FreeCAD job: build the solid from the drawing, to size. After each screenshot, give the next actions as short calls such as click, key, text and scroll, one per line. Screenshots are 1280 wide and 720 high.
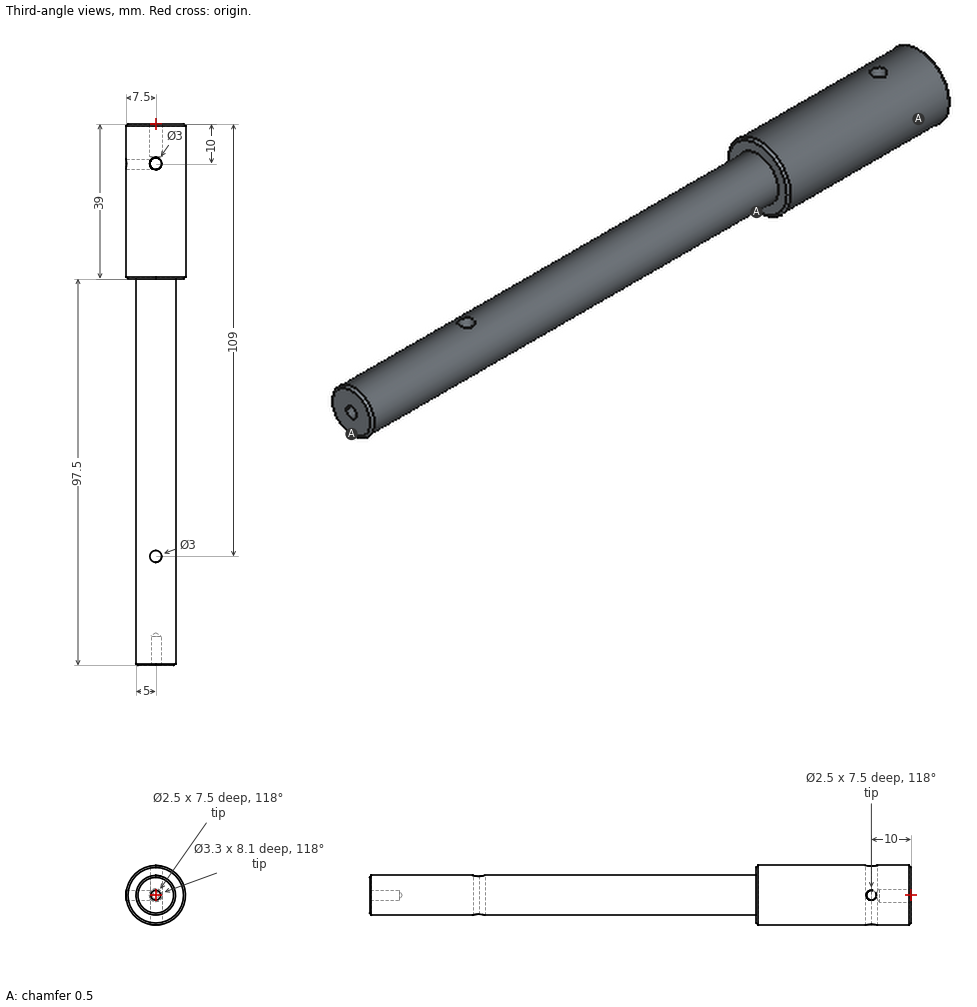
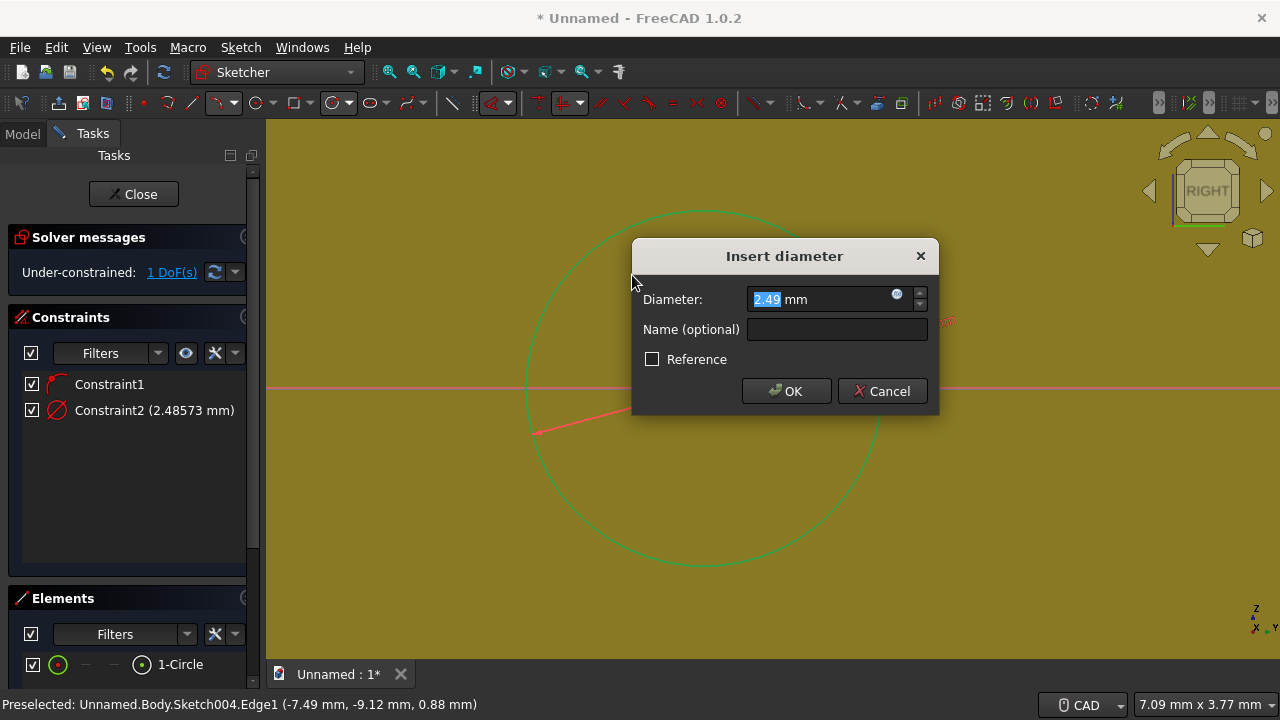
text(2.5)
key(Return)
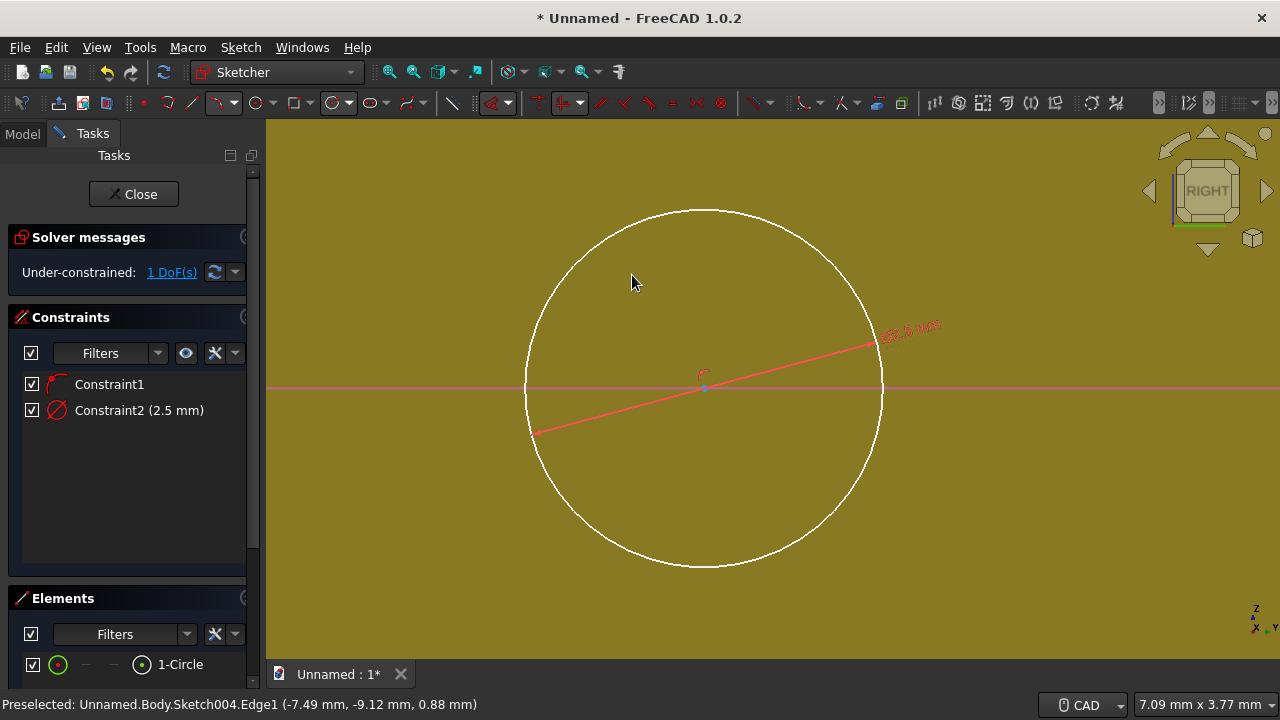
click(704, 388)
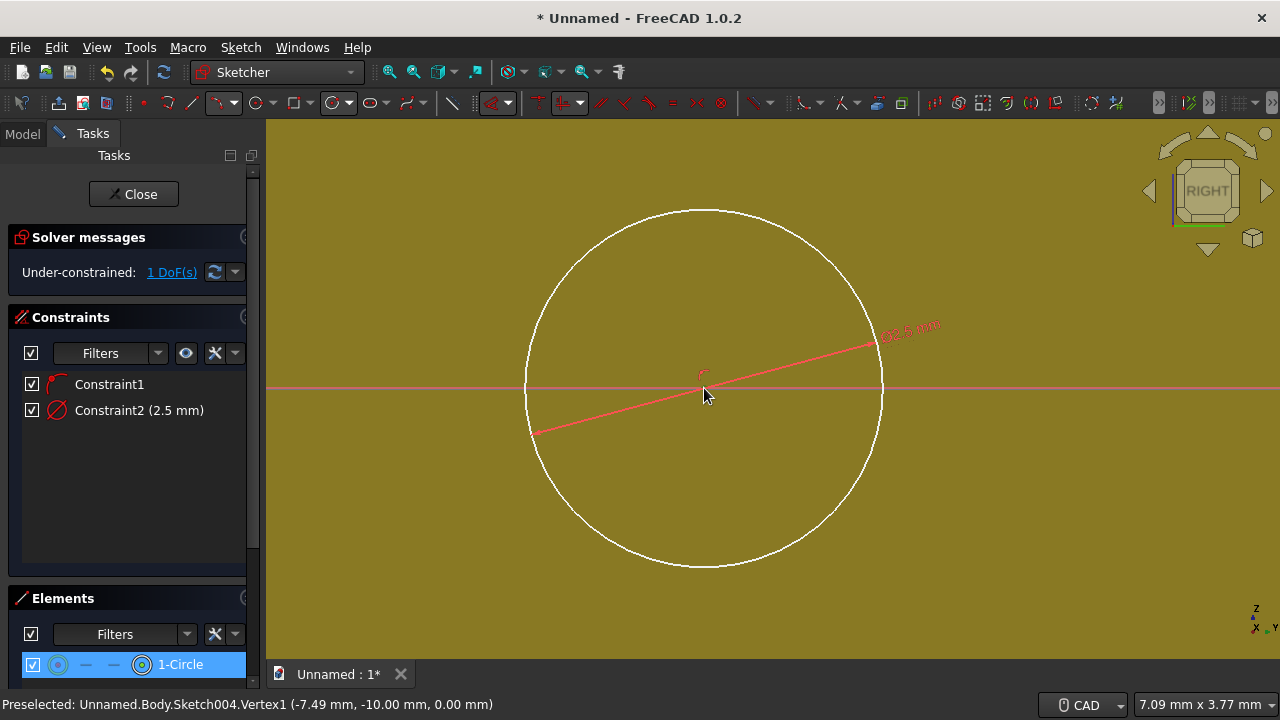
key(l)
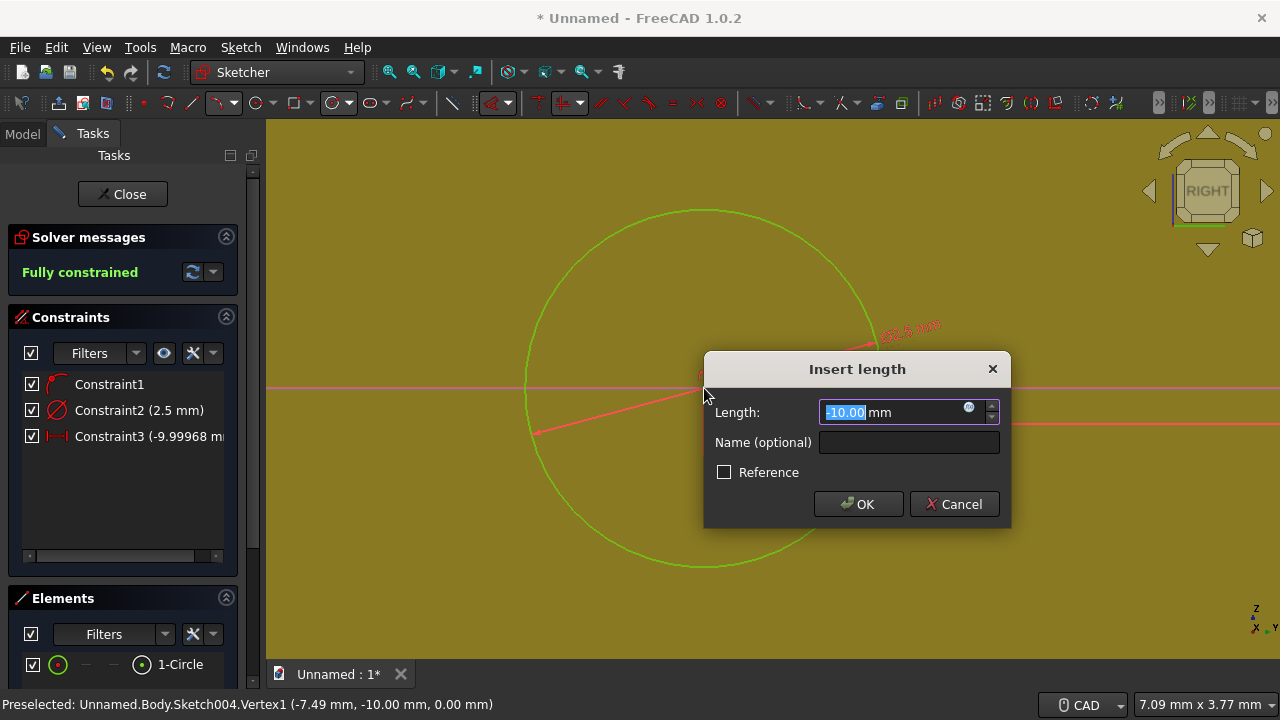
text(-10)
key(Return)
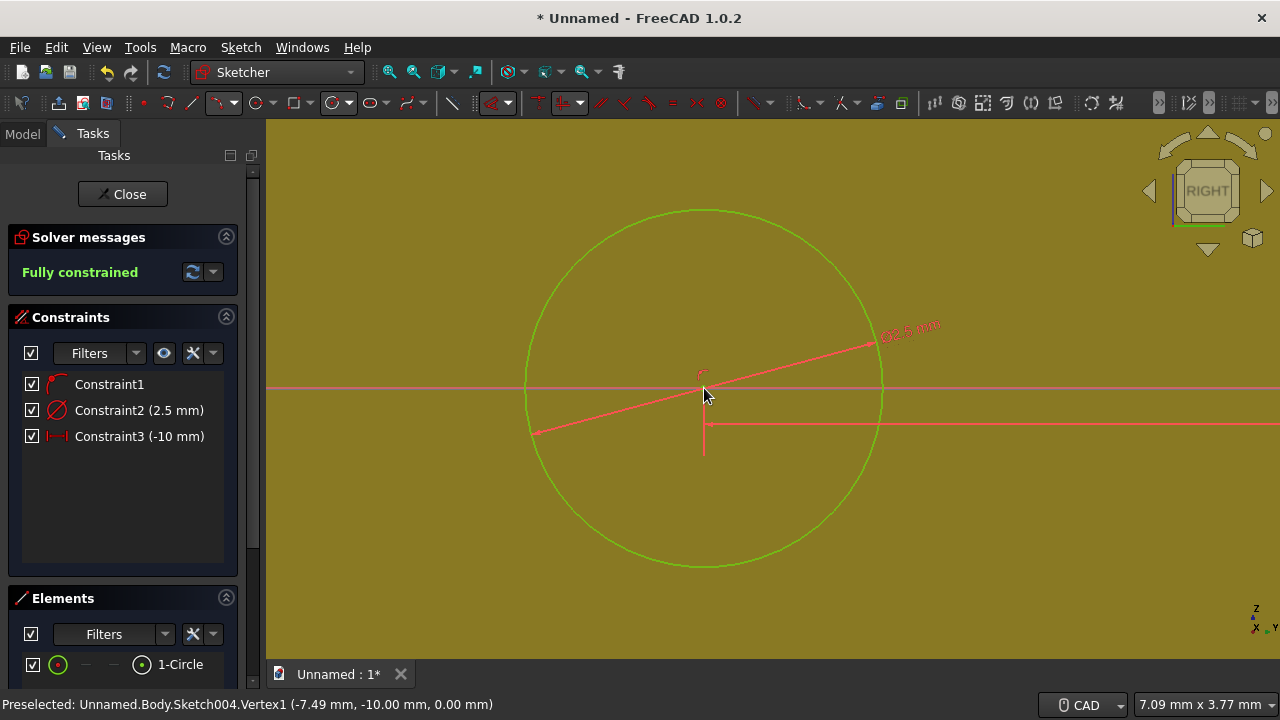
click(123, 194)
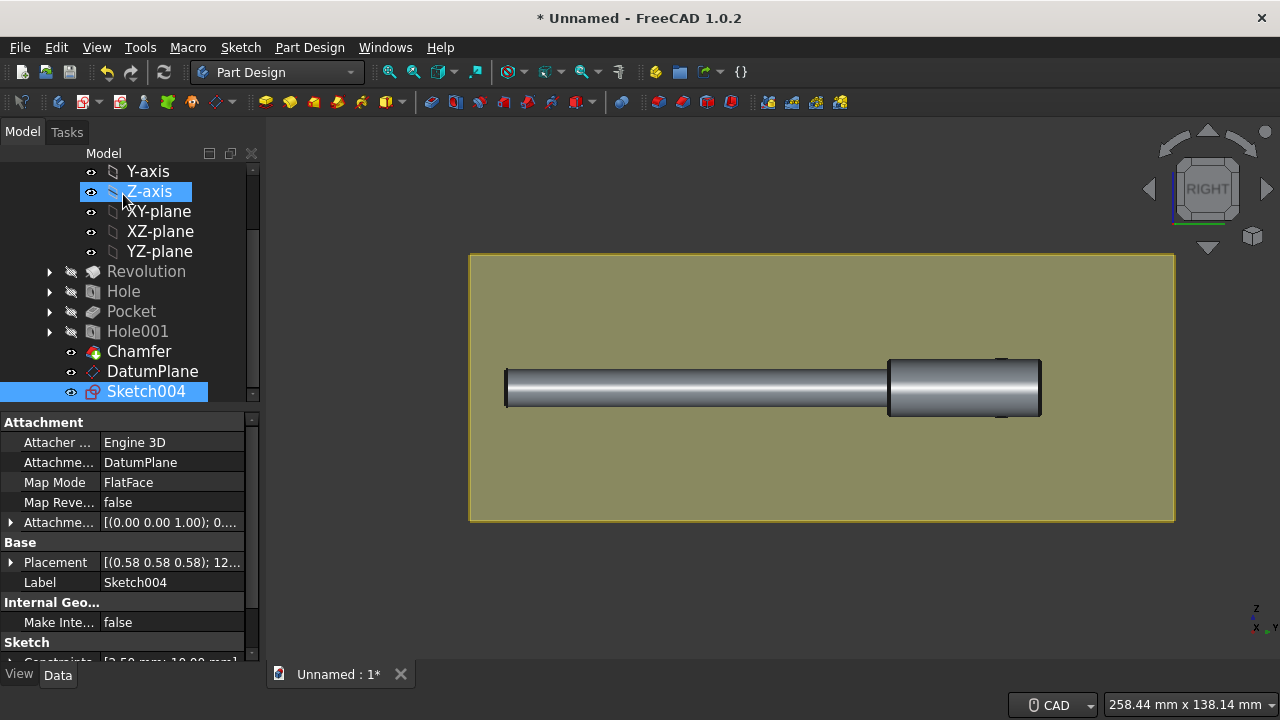
click(456, 102)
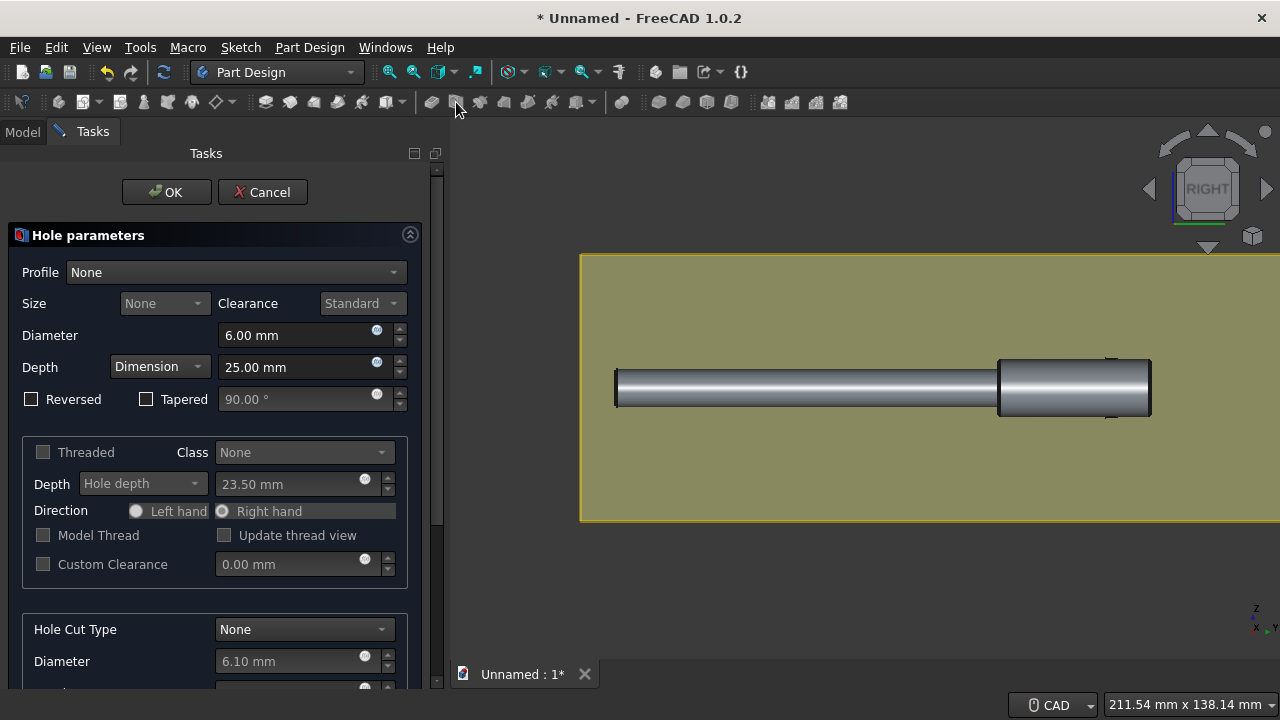
triple_click(305, 335)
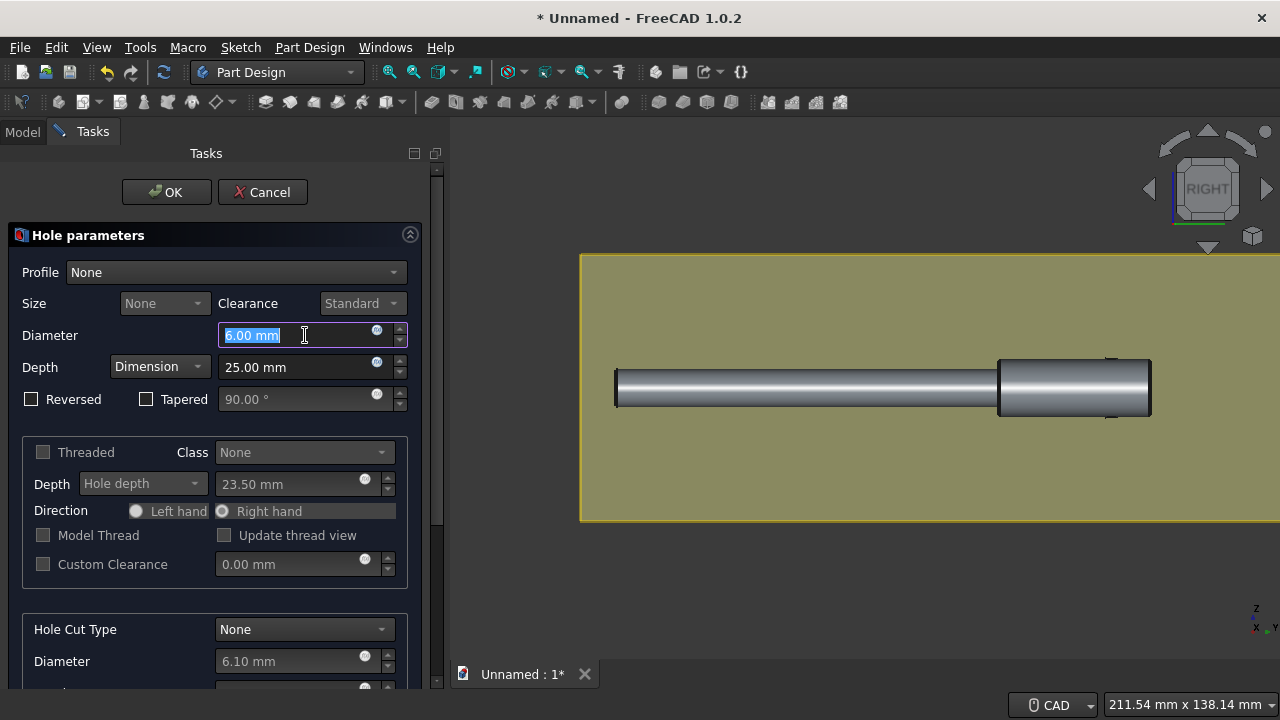
text(2.5)
key(Tab)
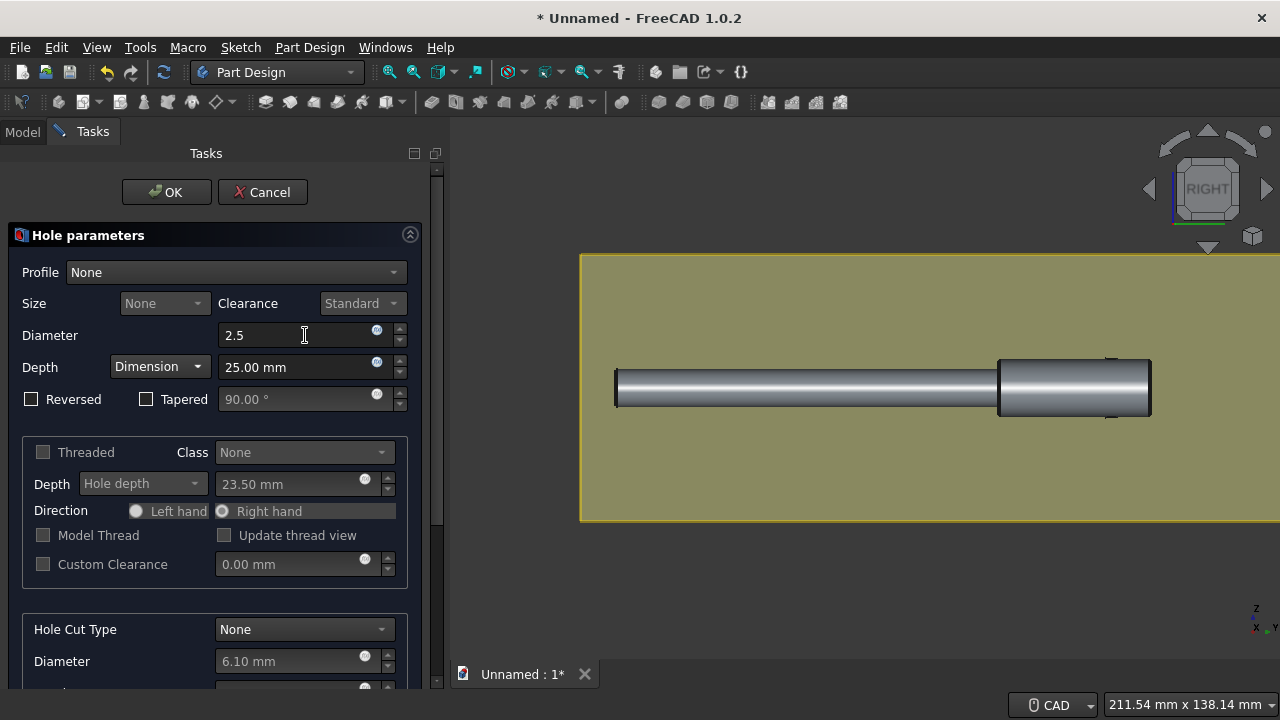
triple_click(305, 367)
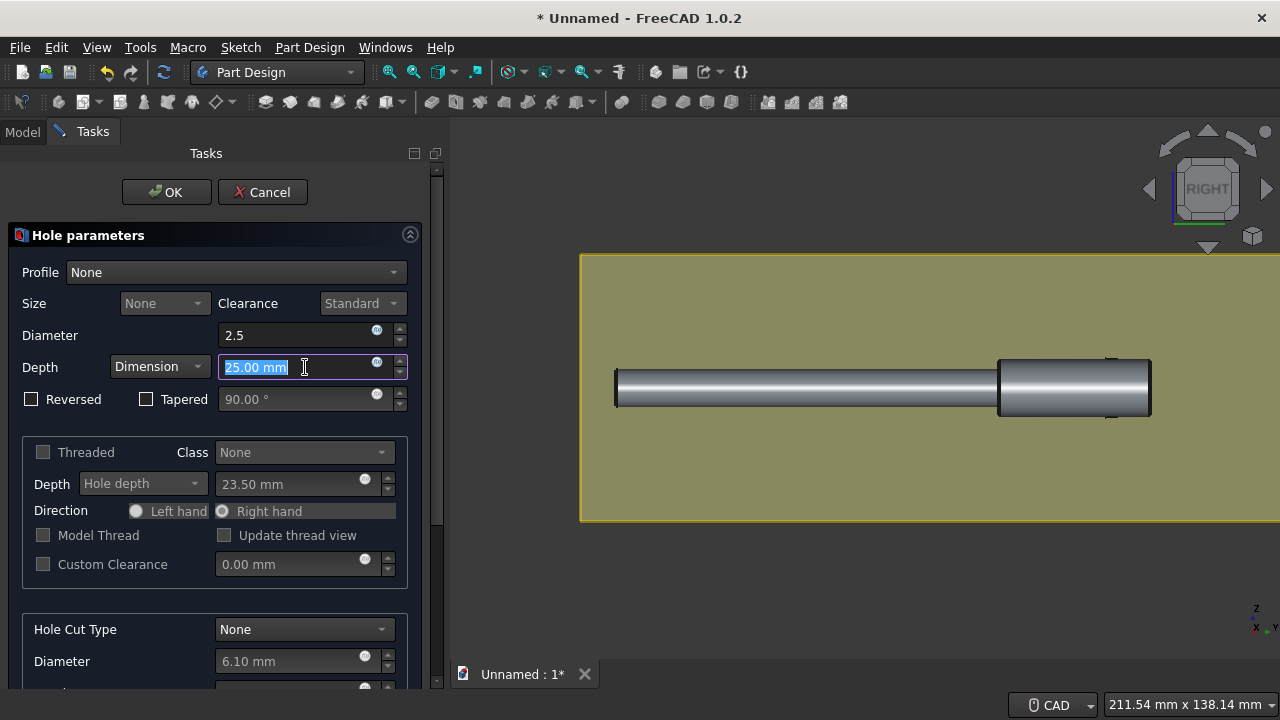
text(7.5)
key(Tab)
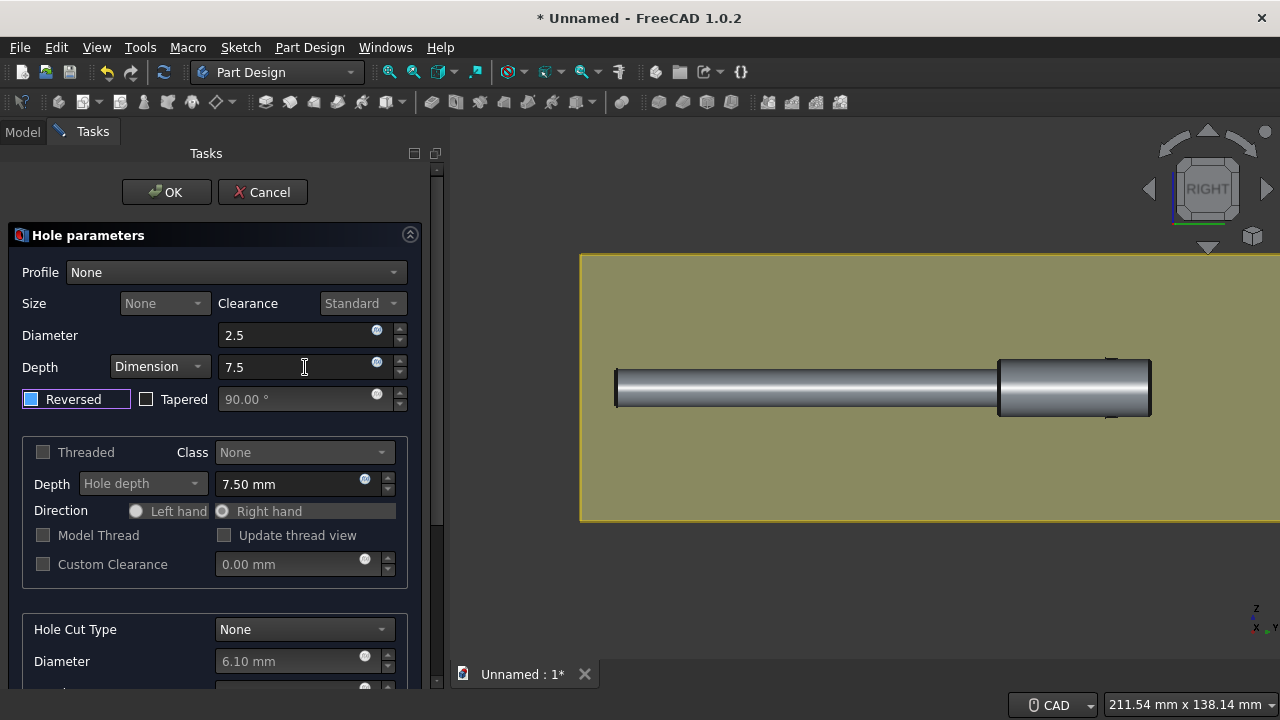
click(30, 399)